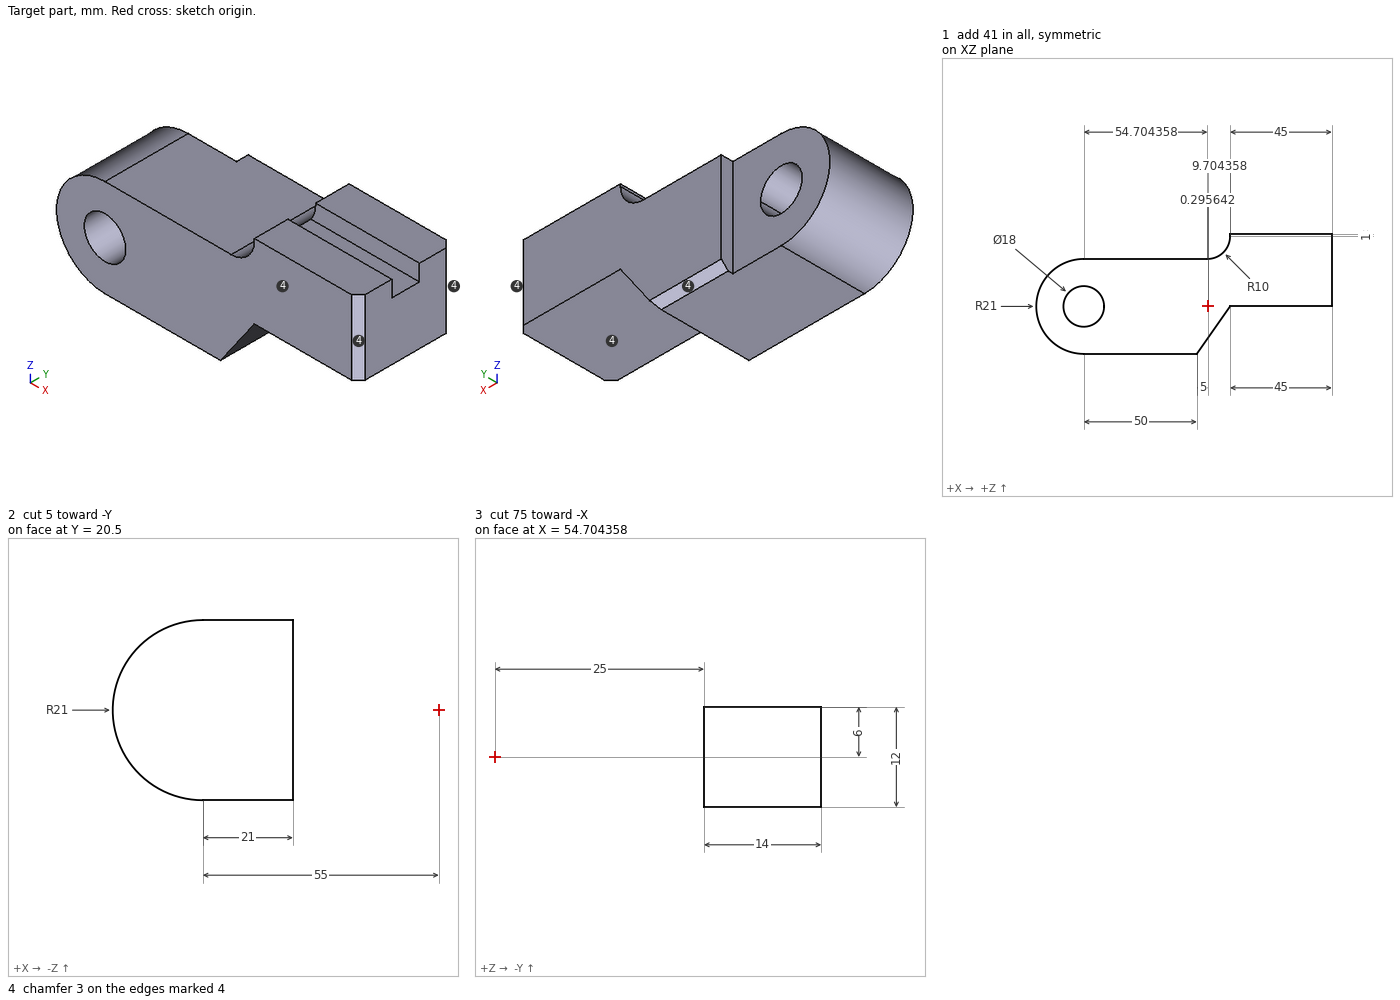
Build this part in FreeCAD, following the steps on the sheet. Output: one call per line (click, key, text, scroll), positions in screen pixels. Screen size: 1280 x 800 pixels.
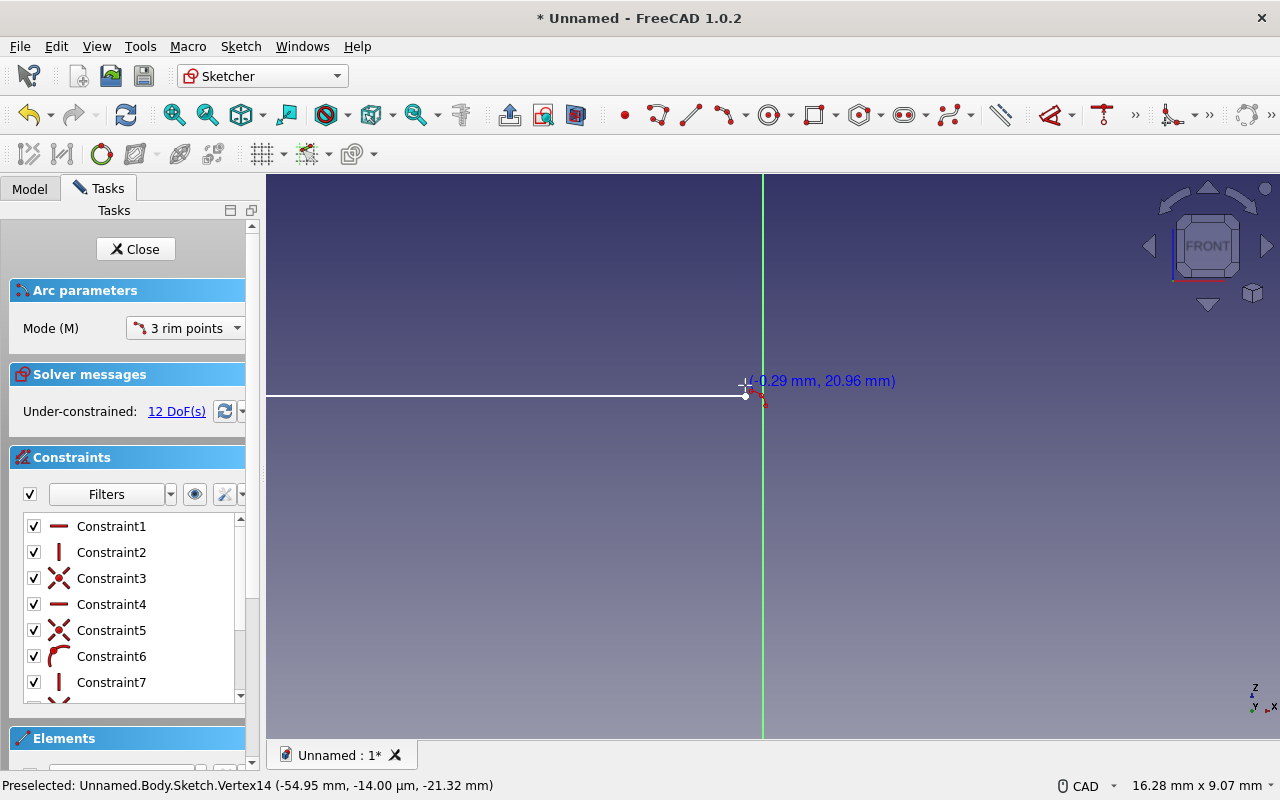
scroll(753, 385, down, 13)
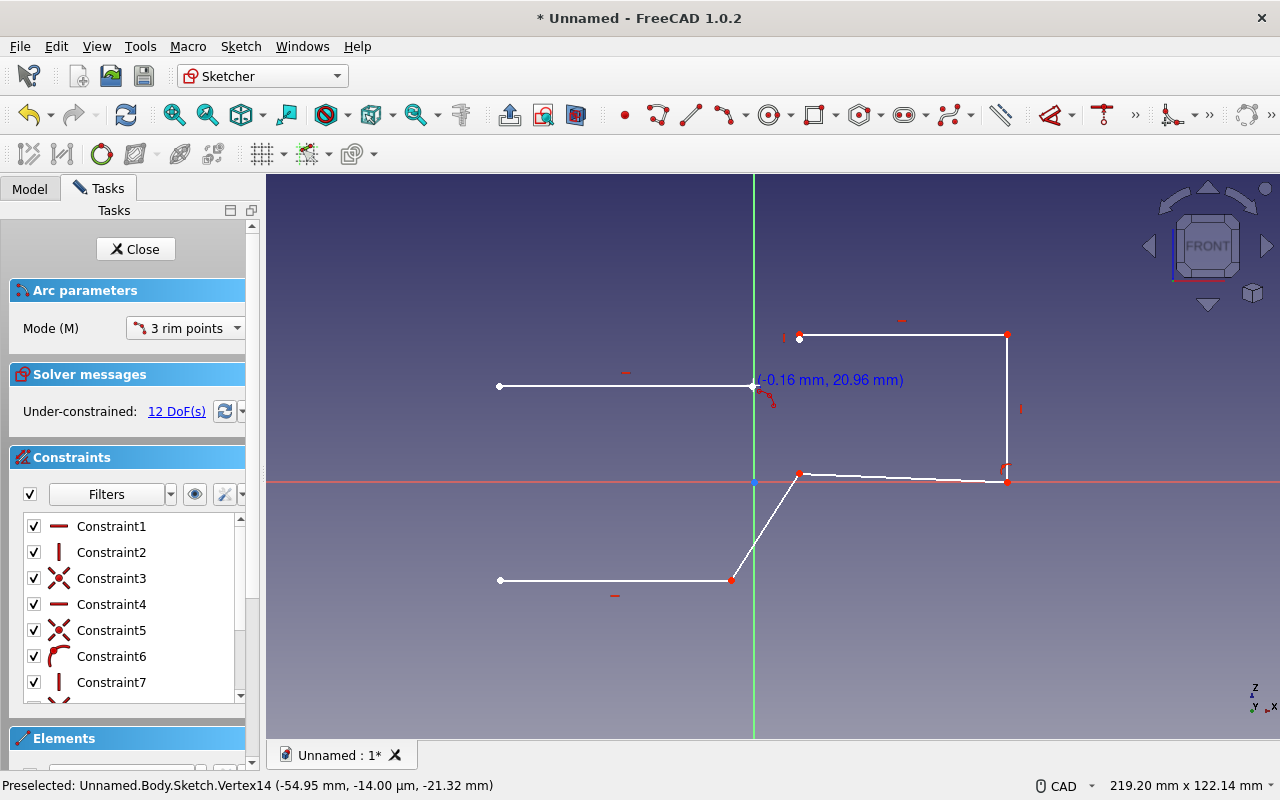
scroll(799, 339, up, 10)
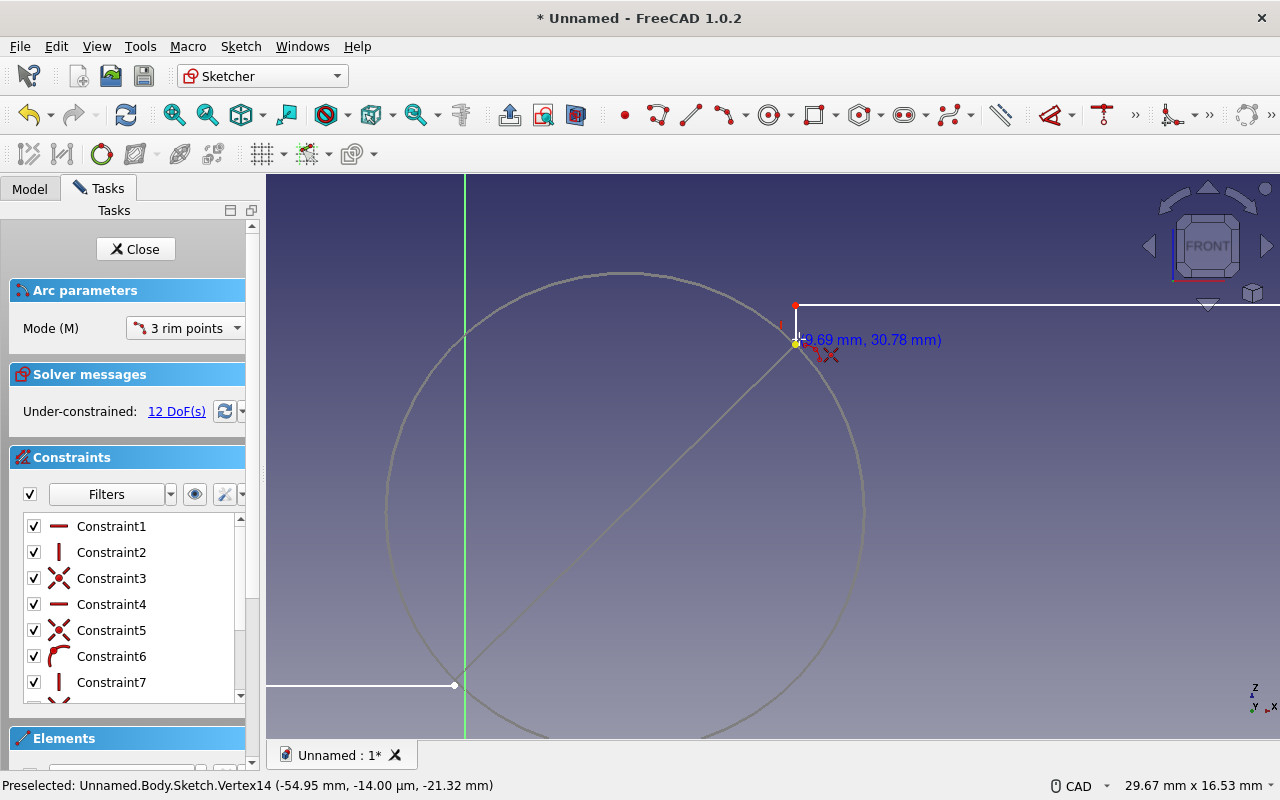
click(796, 345)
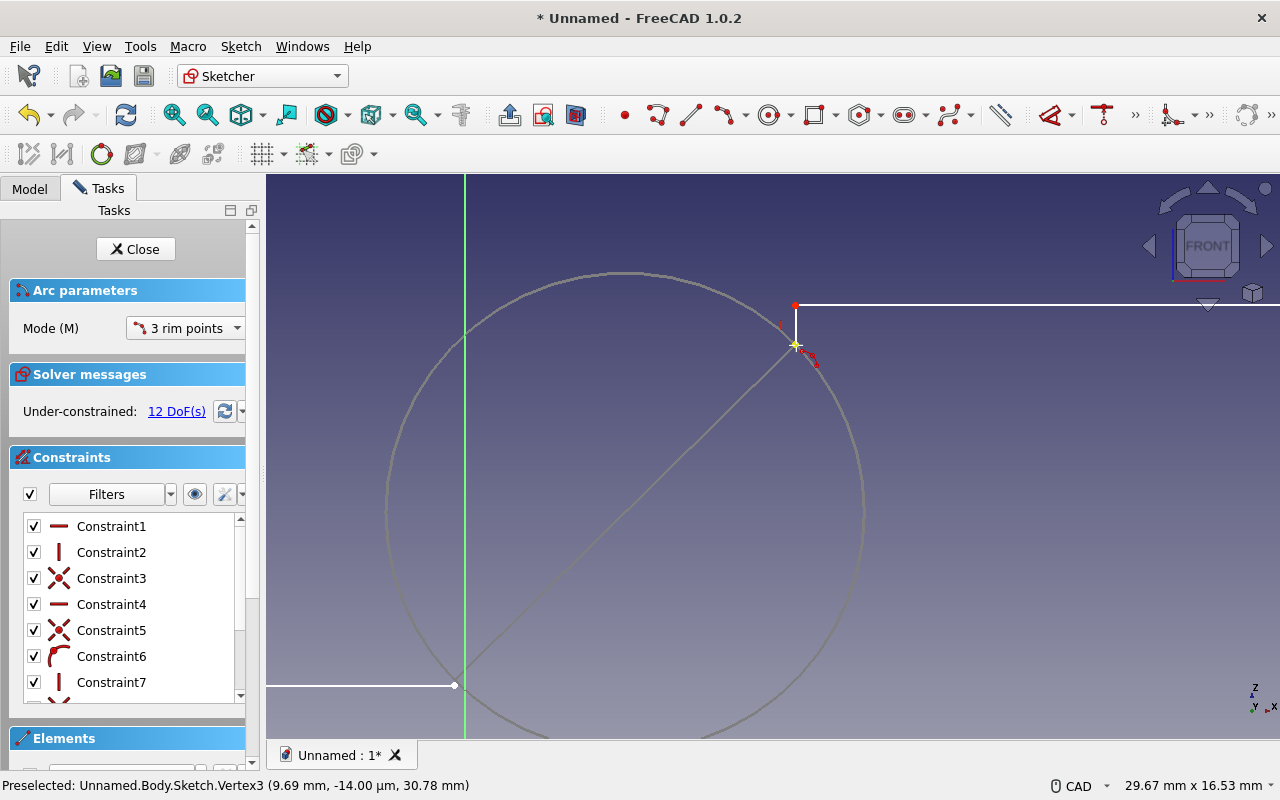
scroll(799, 339, down, 10)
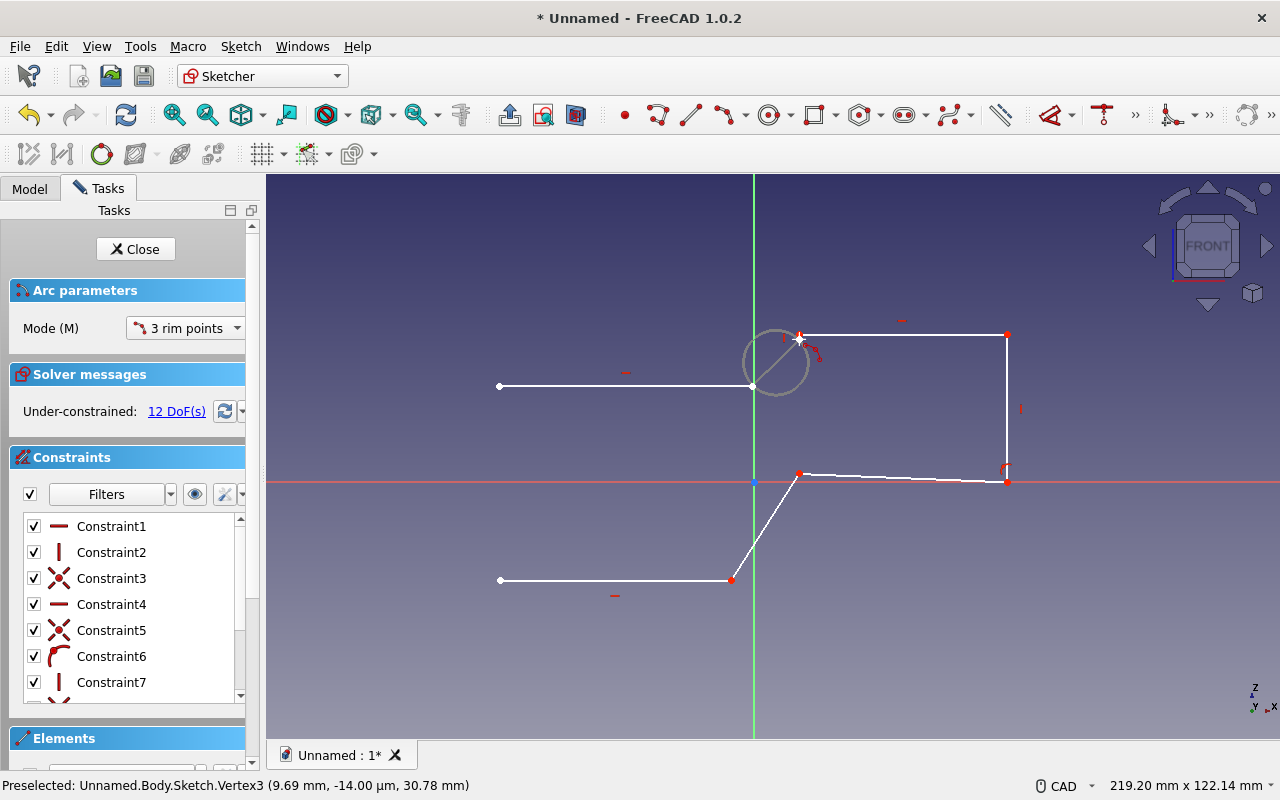
click(786, 372)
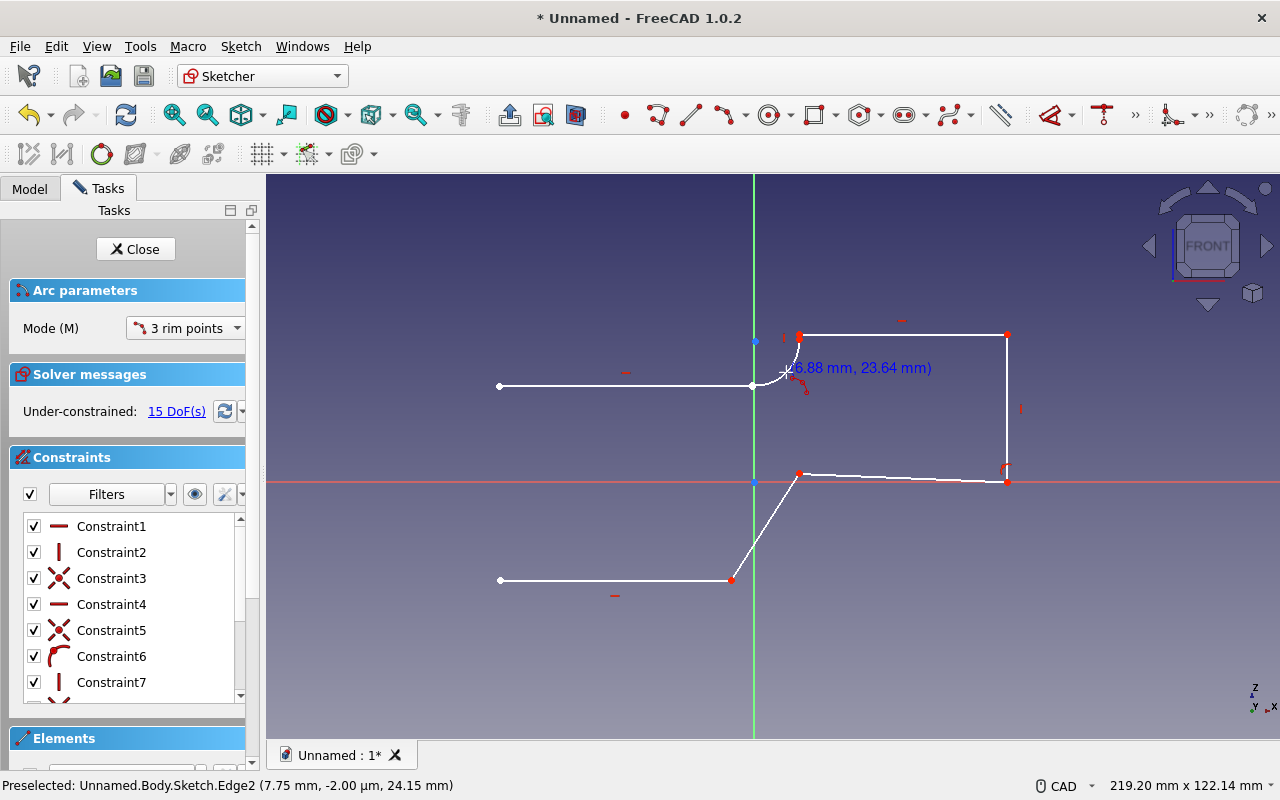
click(500, 581)
click(500, 386)
click(407, 452)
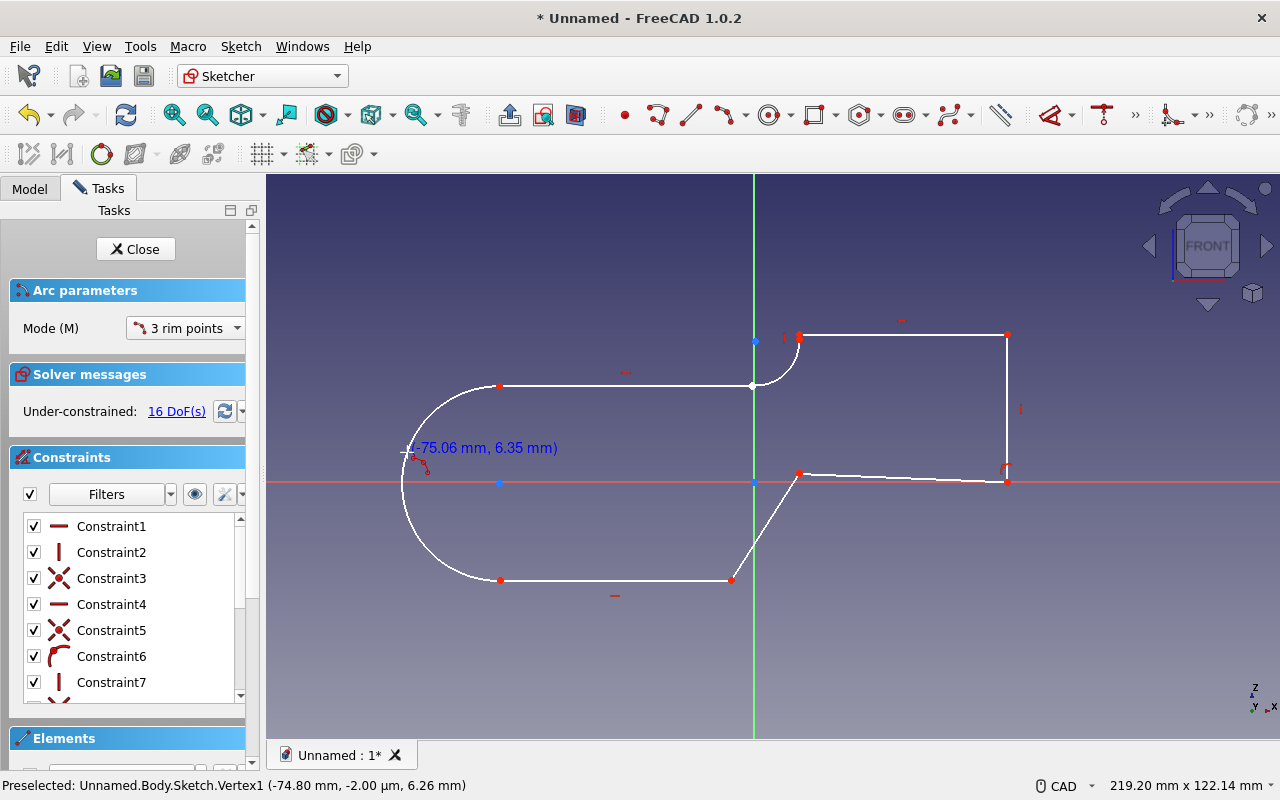
click(768, 116)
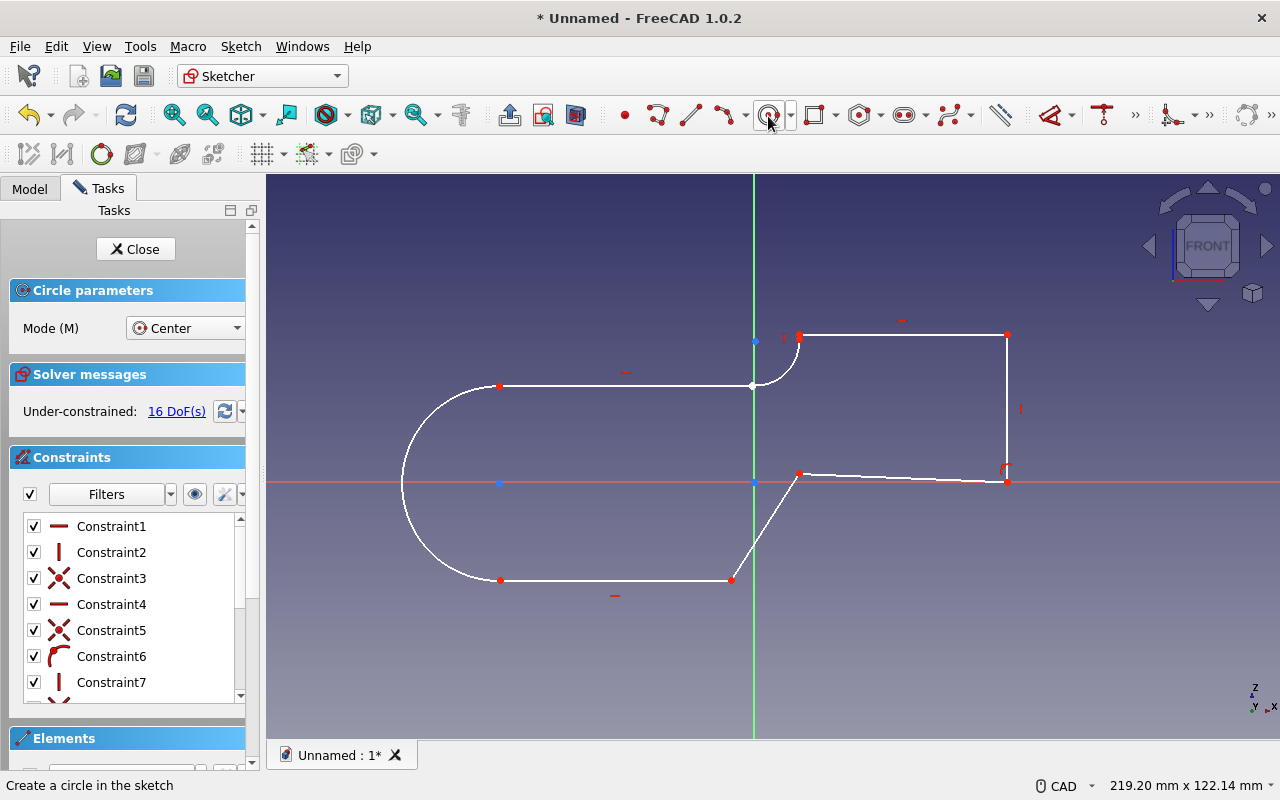
click(500, 482)
click(529, 453)
key(Escape)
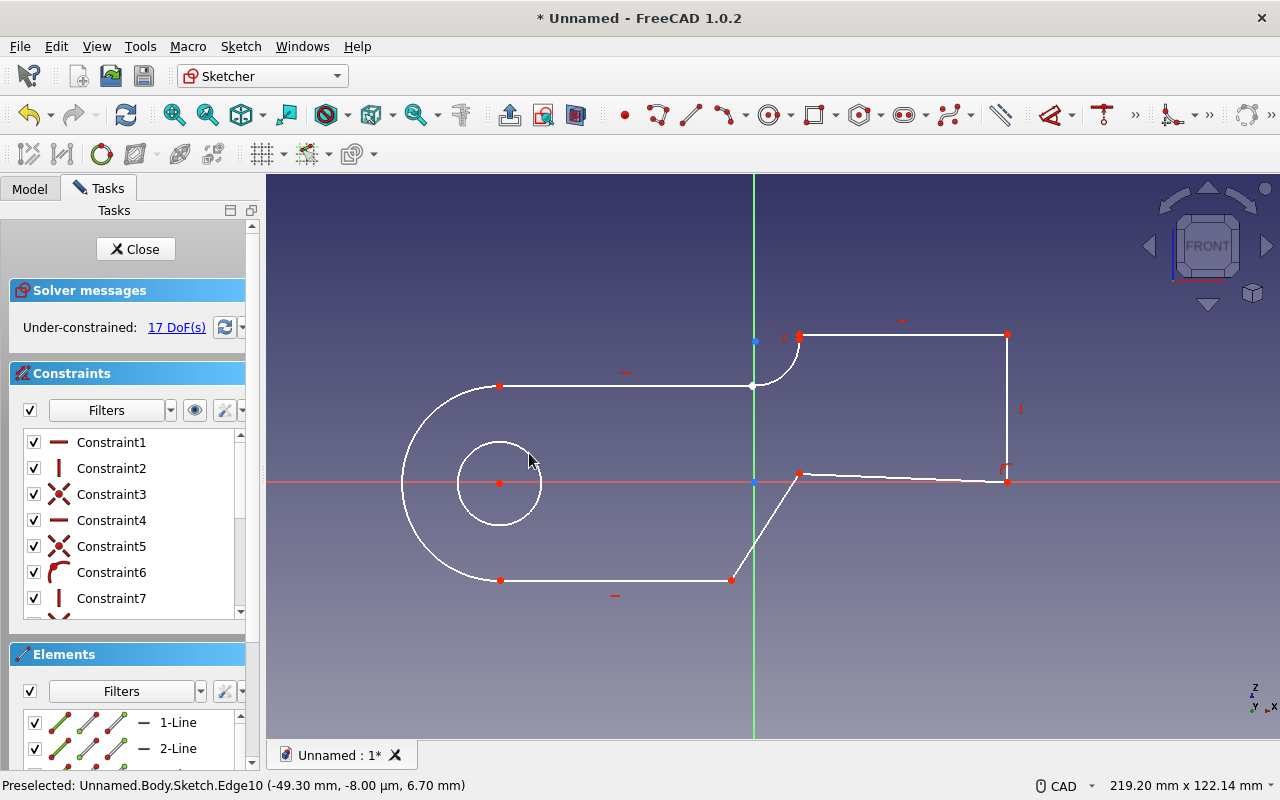
click(576, 386)